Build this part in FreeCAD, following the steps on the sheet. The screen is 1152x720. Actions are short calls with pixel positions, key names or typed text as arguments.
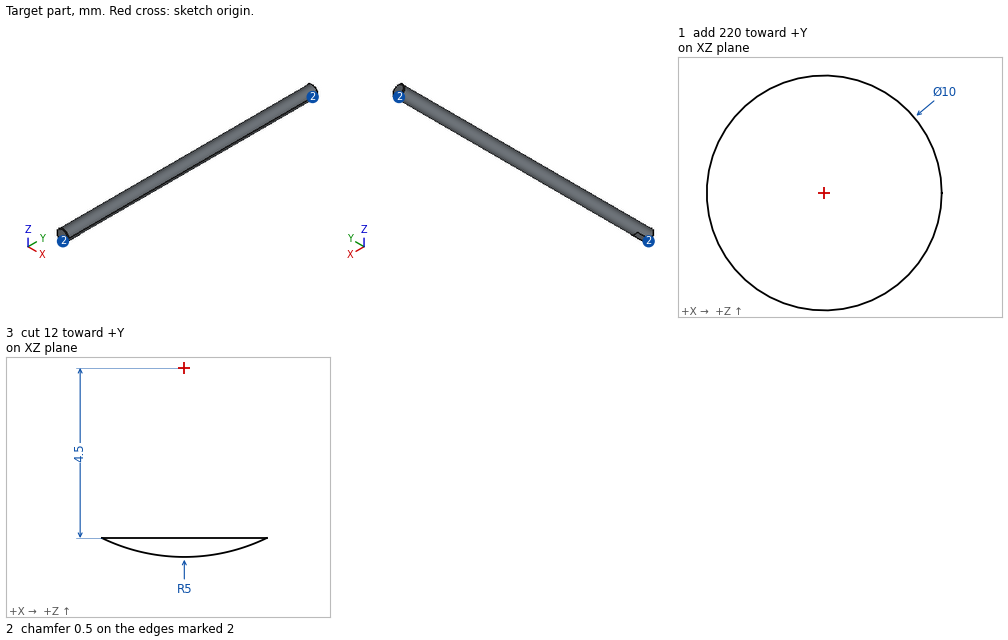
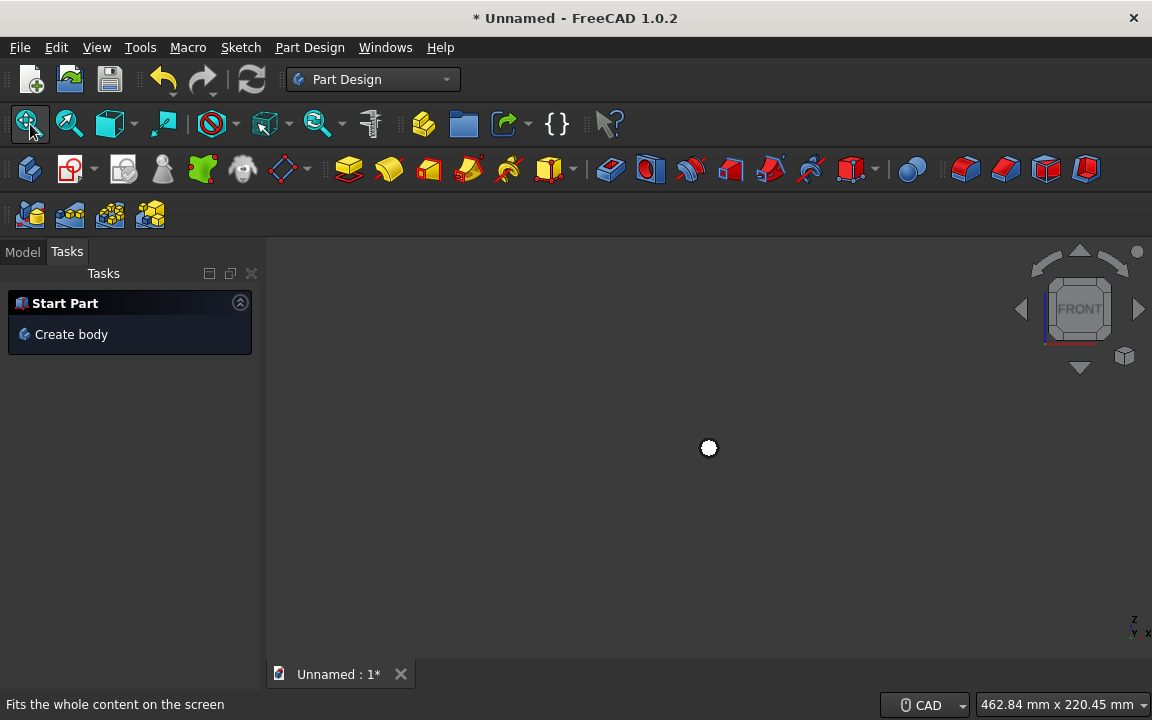
key(2)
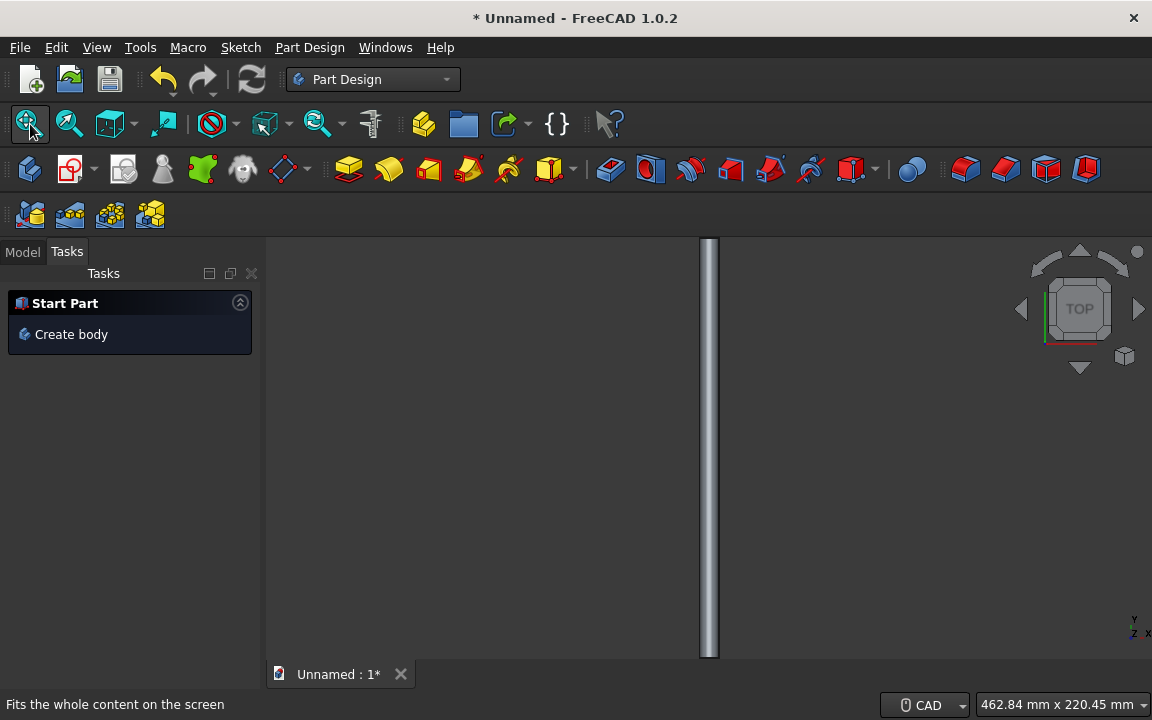
key(v)
key(f)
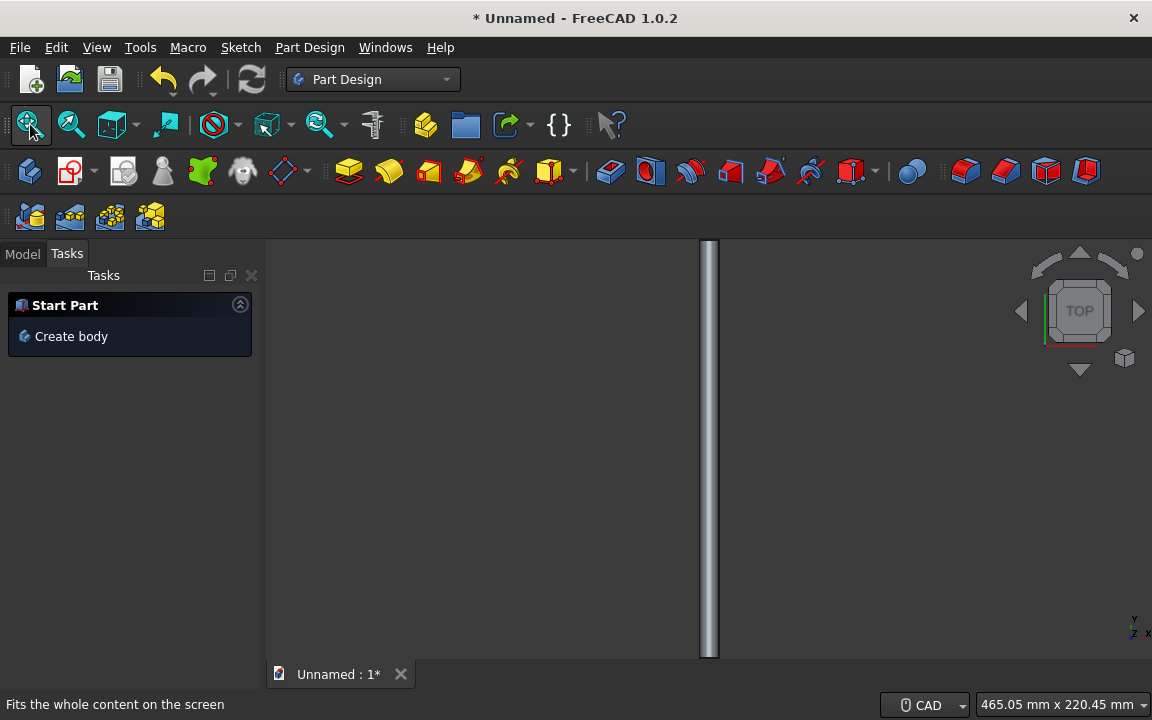
click(70, 172)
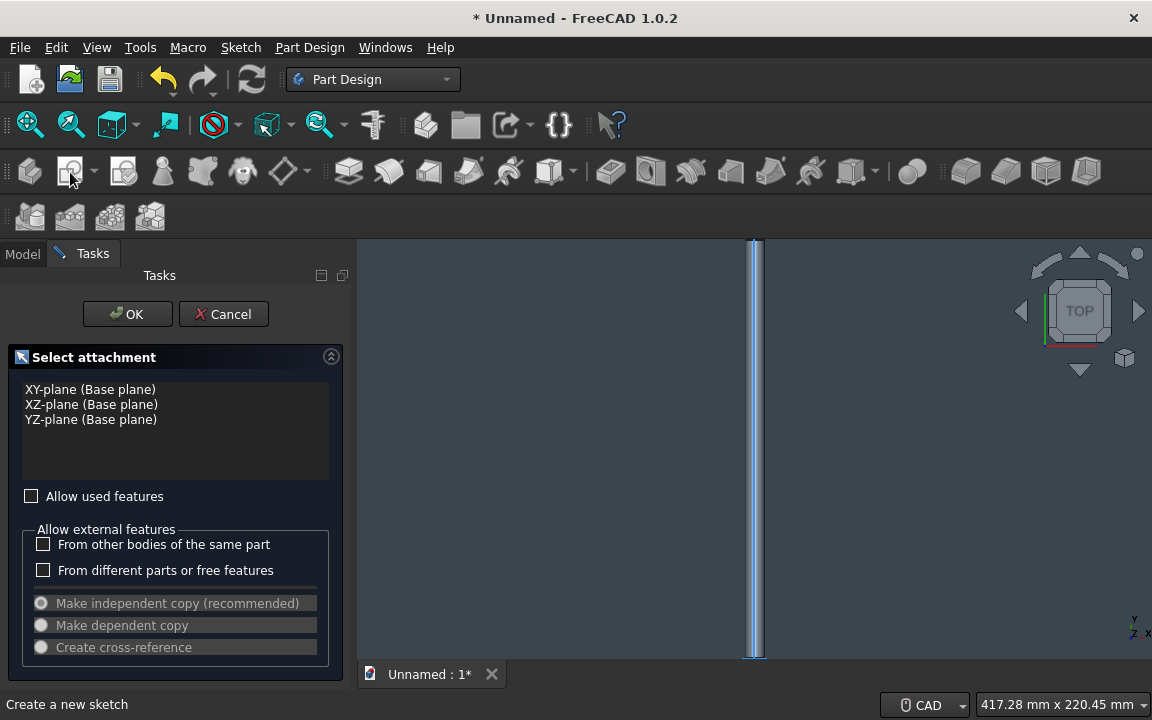
click(82, 404)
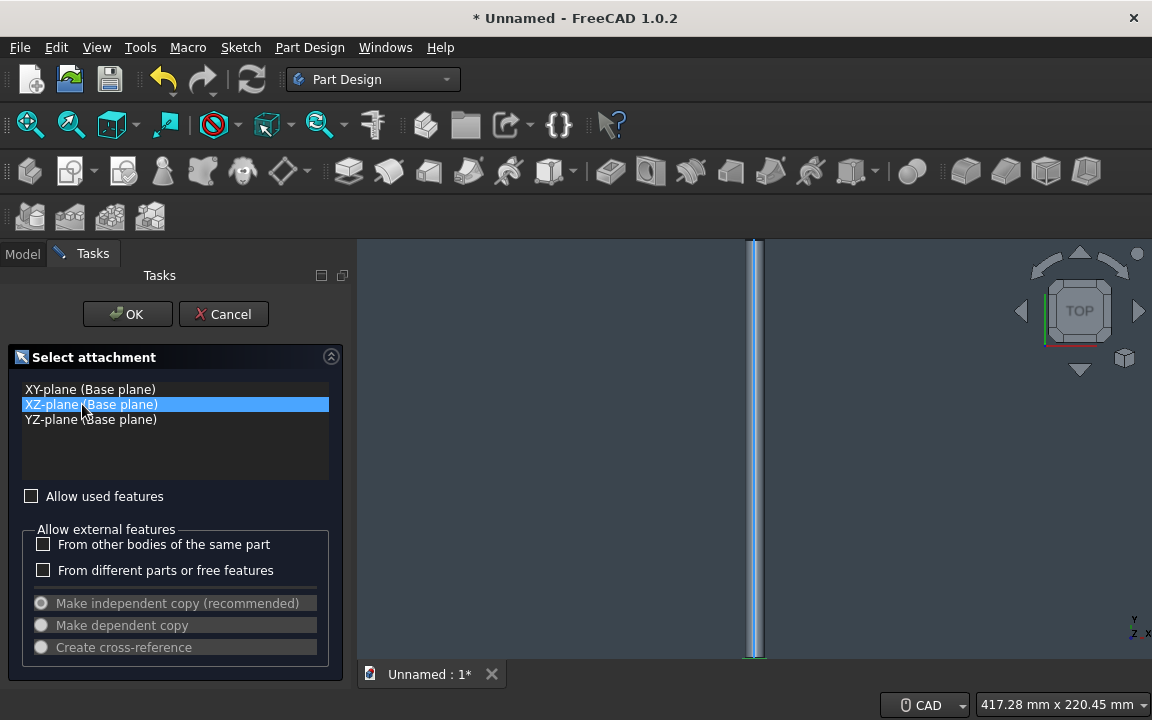
click(128, 314)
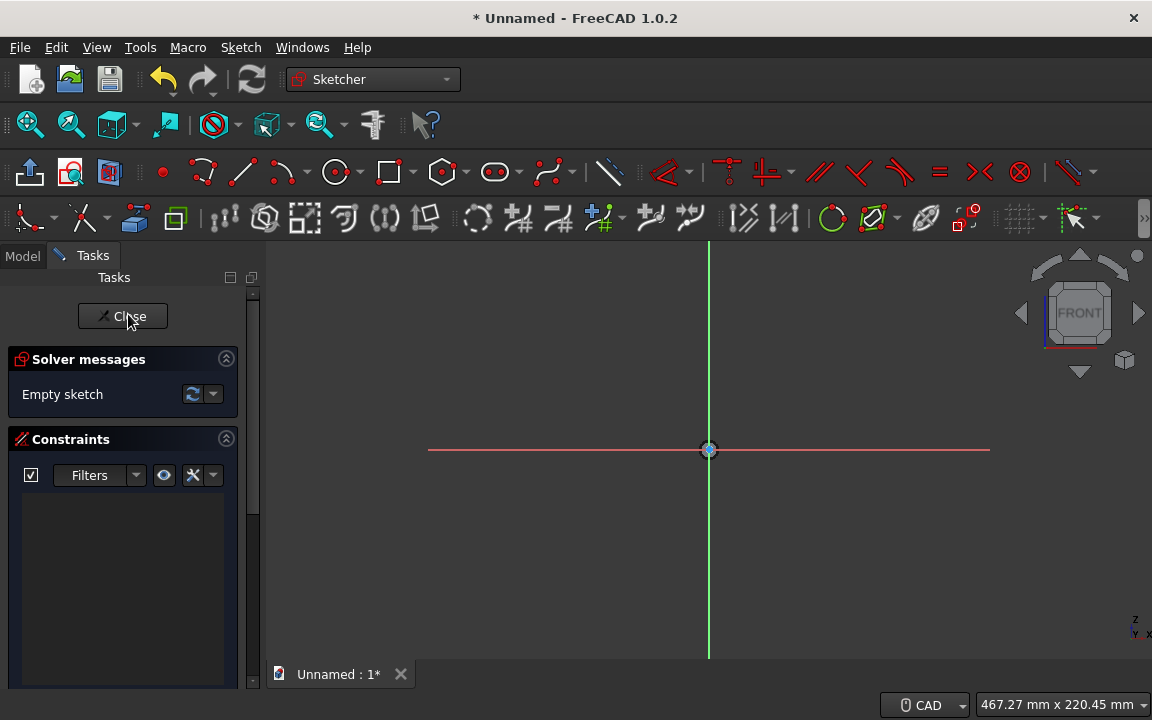
scroll(713, 455, up, 15)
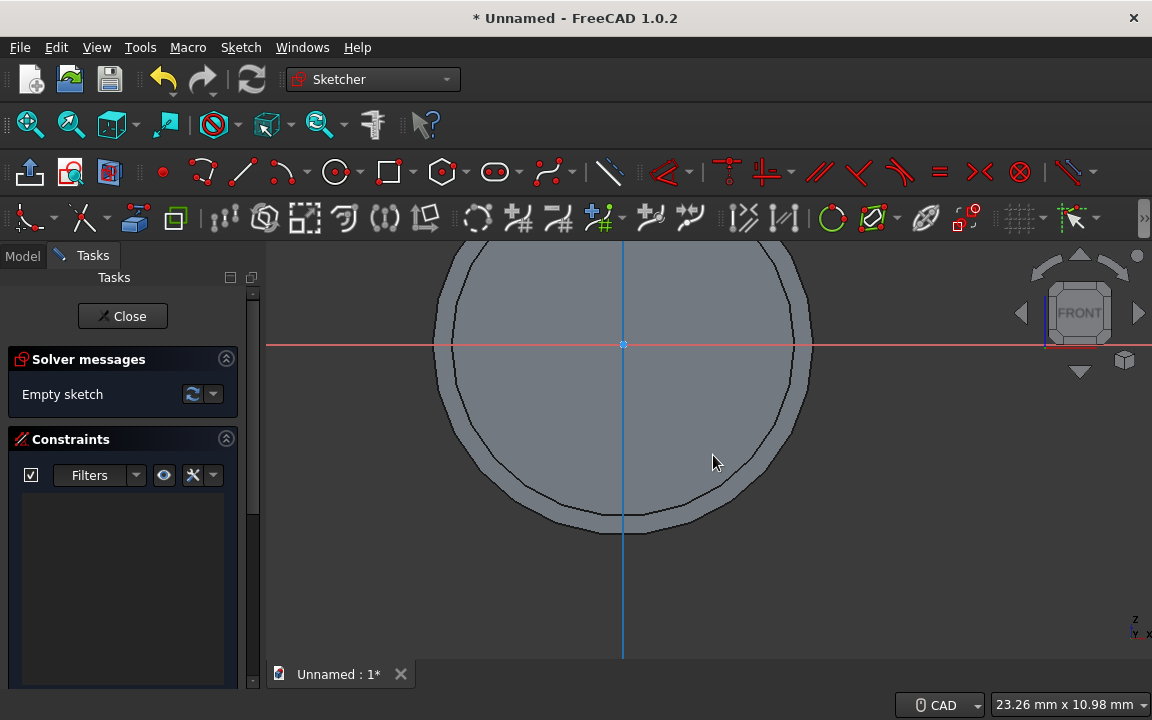
key(g)
key(l)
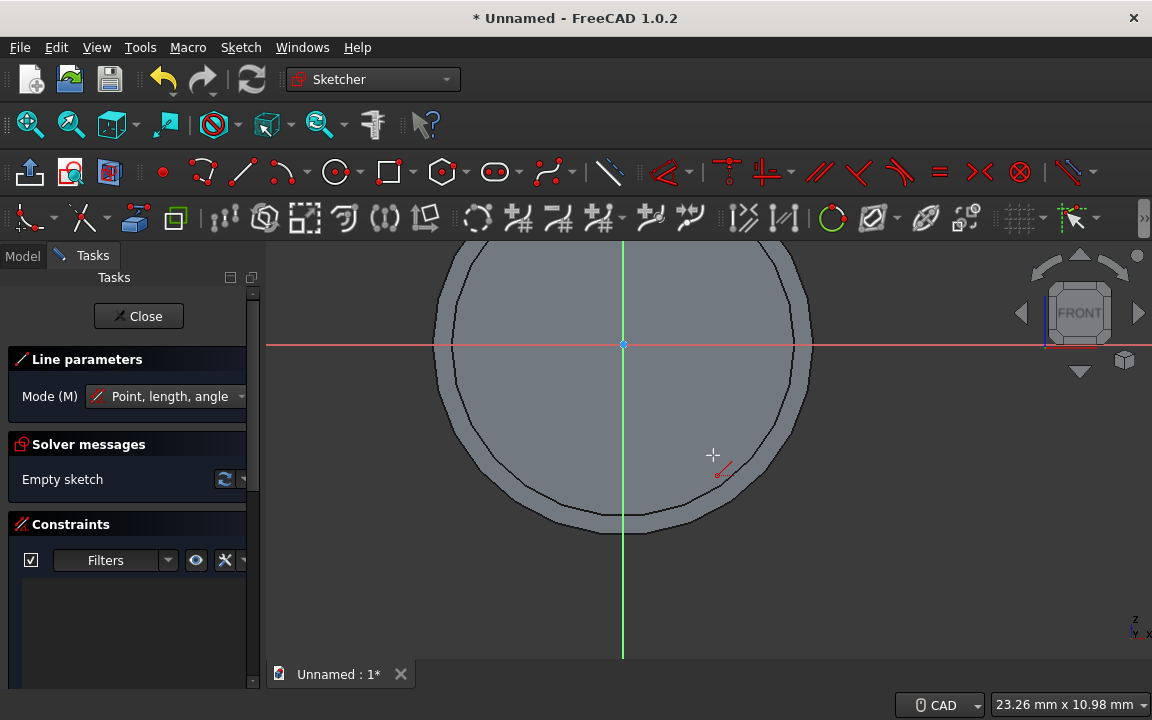
click(540, 516)
click(706, 516)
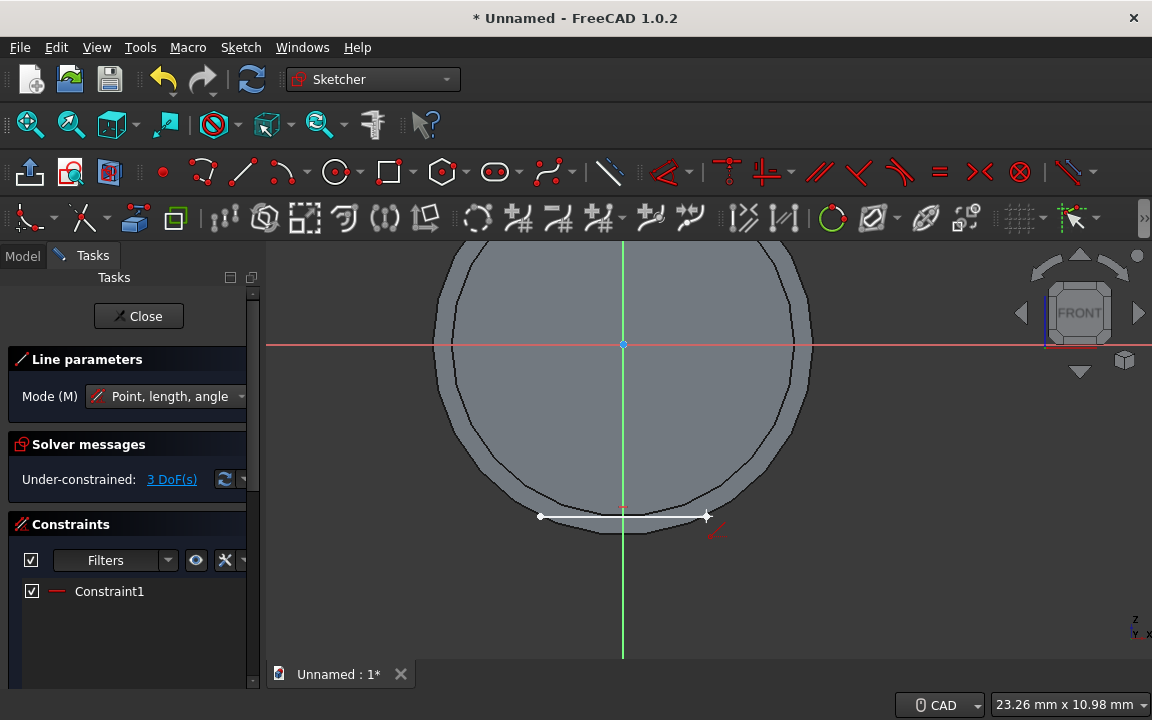
key(g)
key(3)
key(a)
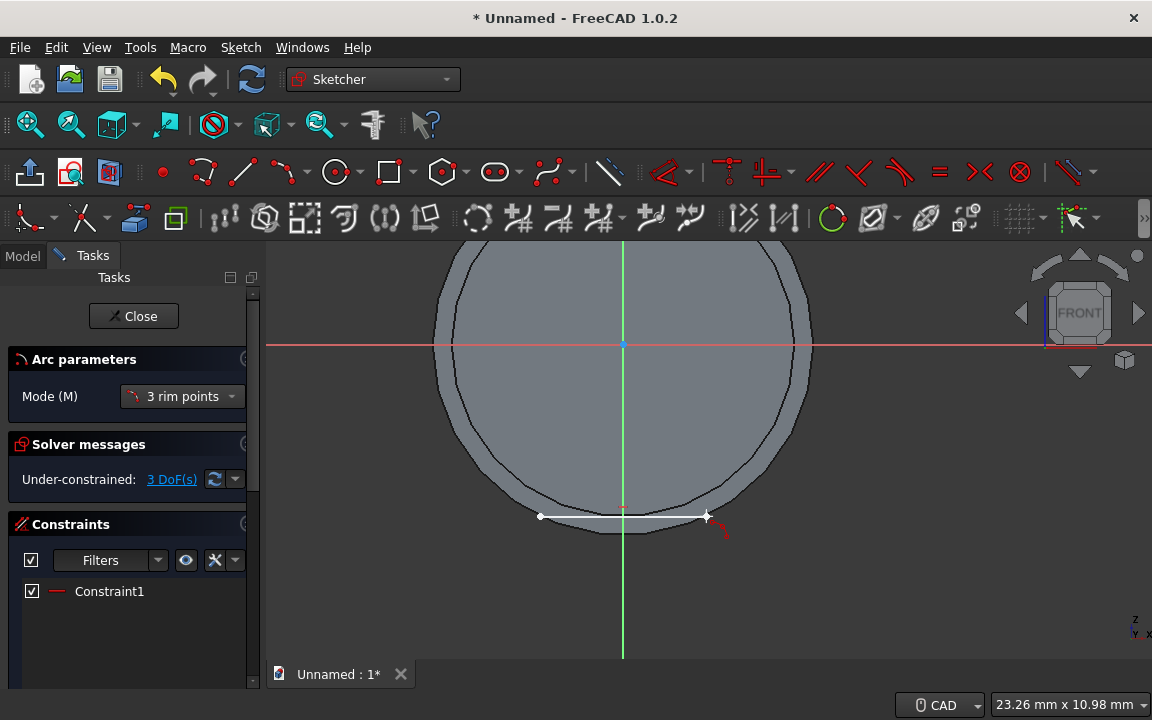
click(706, 517)
click(540, 517)
click(606, 534)
key(Escape)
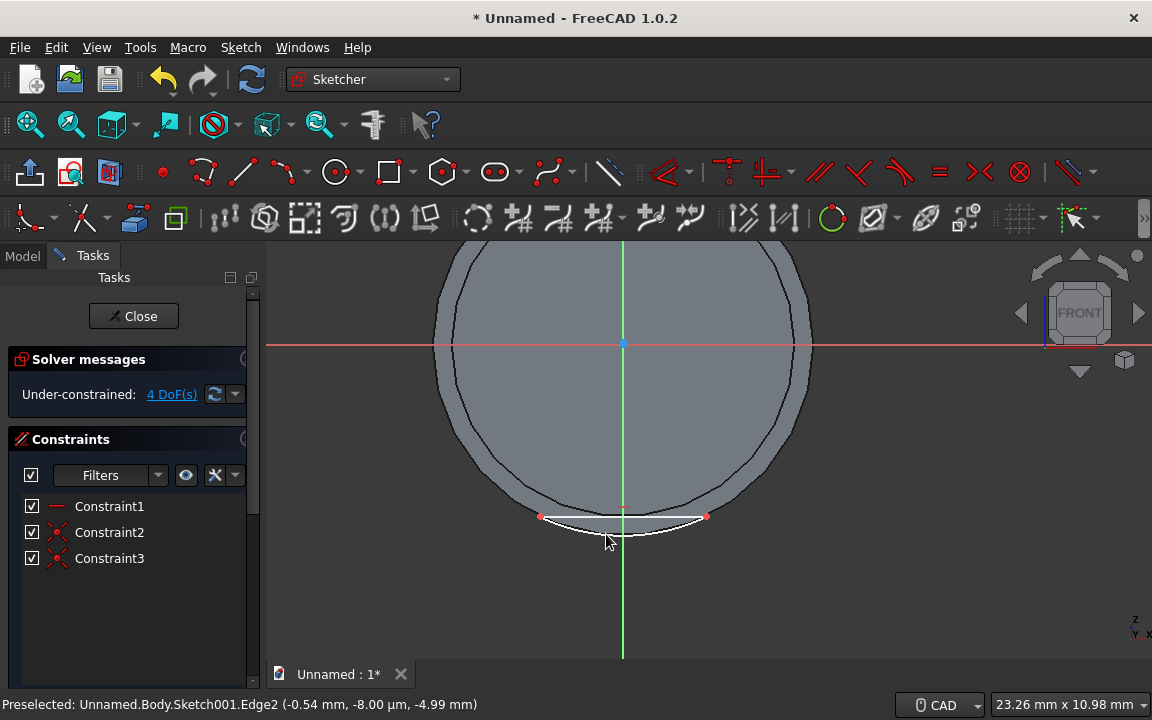
drag(613, 333, 633, 355)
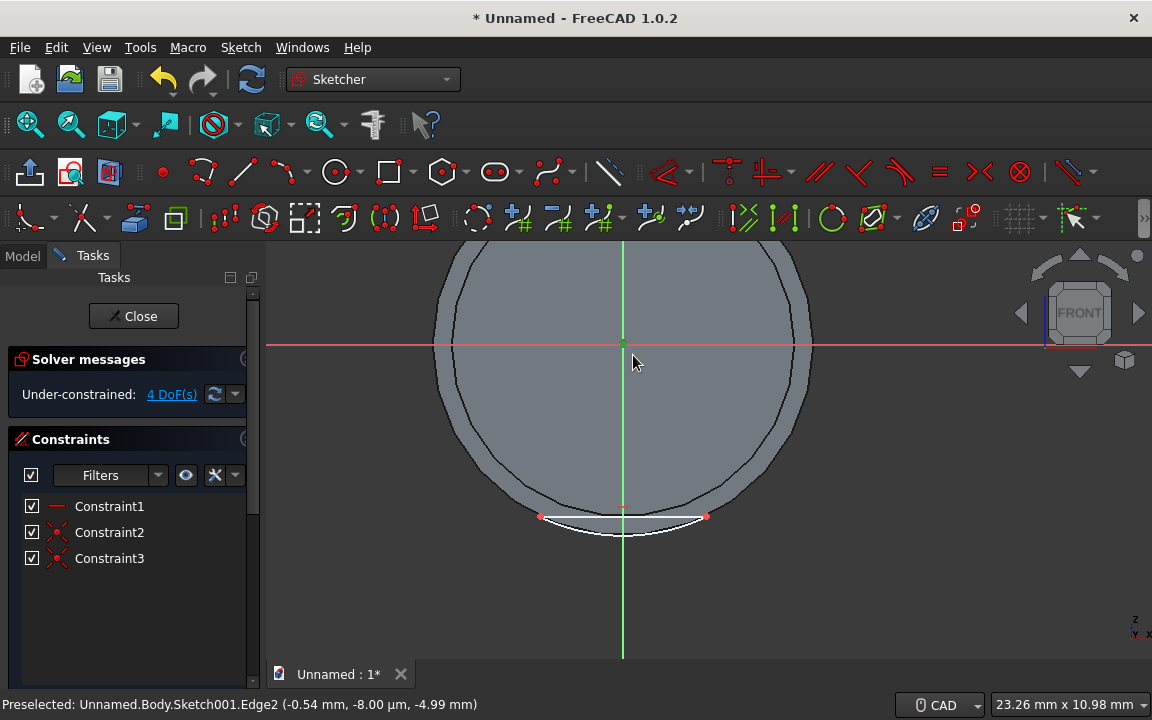
click(728, 172)